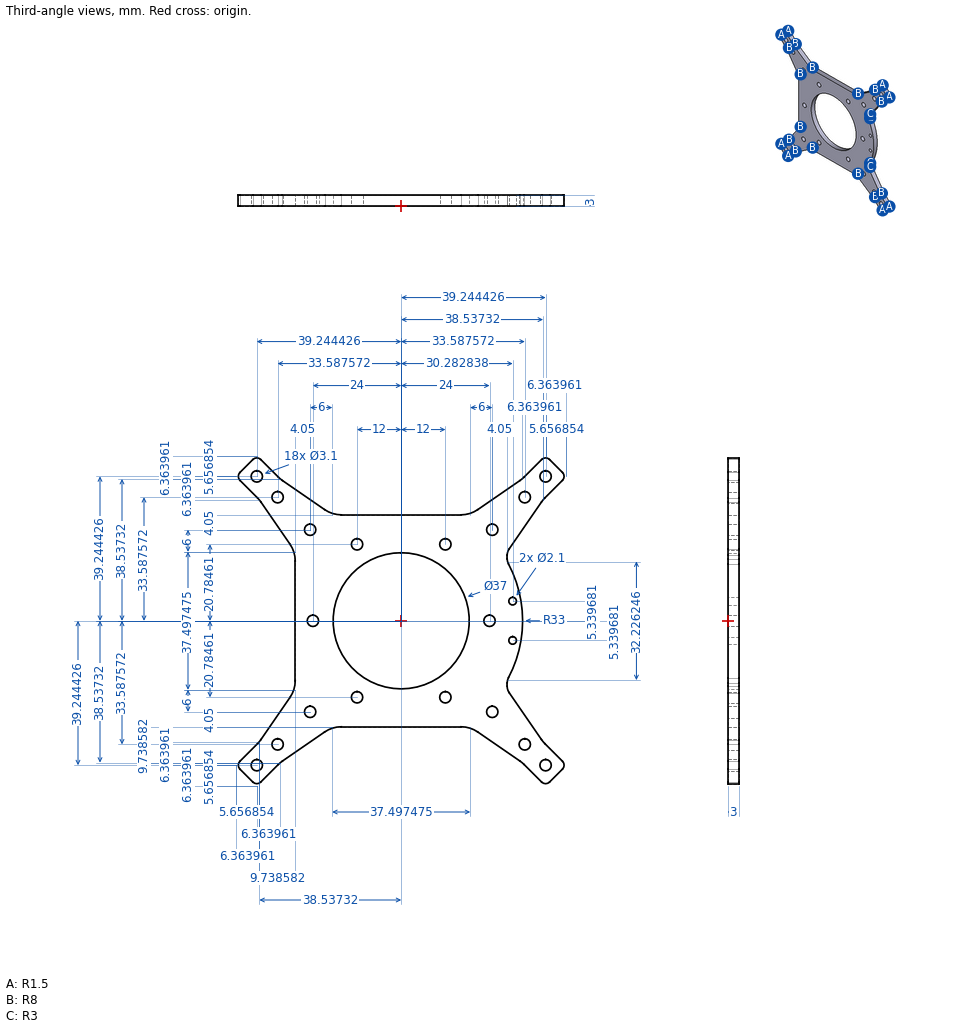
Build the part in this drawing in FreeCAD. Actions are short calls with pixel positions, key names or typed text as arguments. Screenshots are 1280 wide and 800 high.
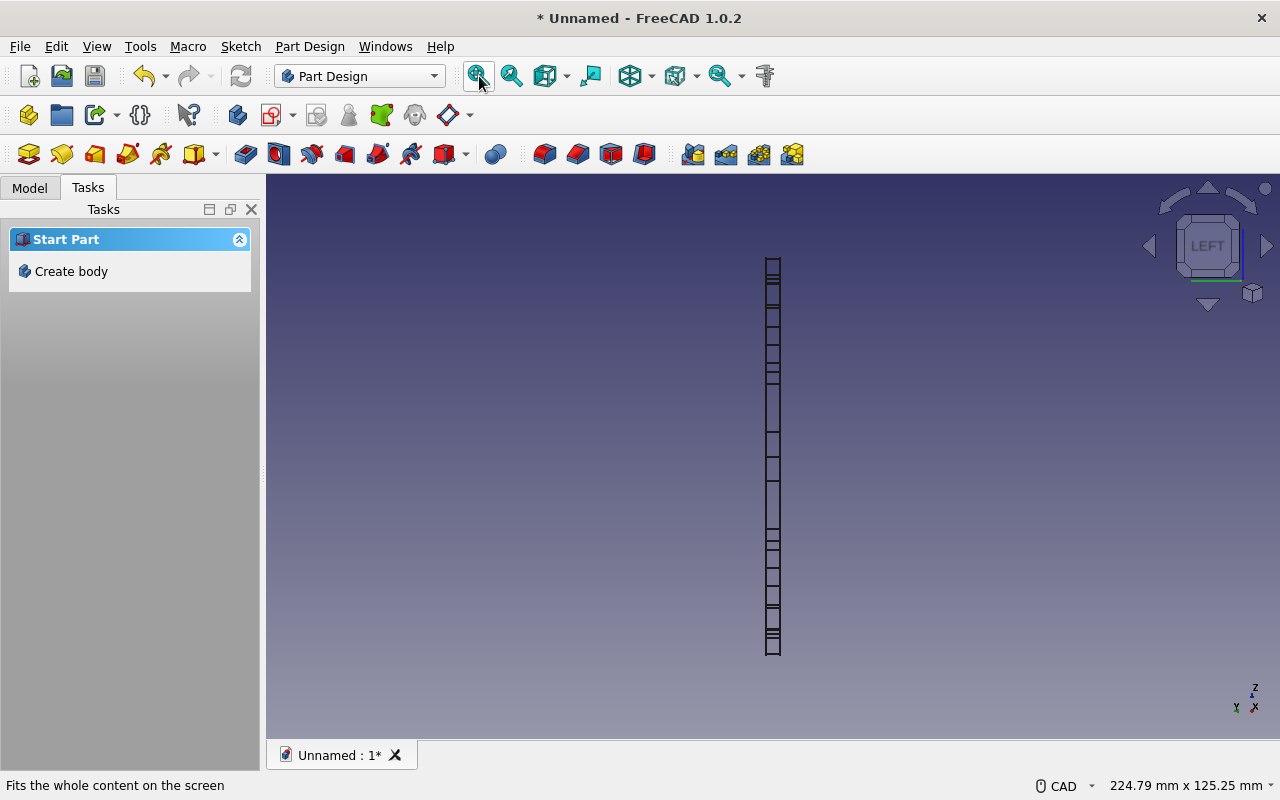
key(0)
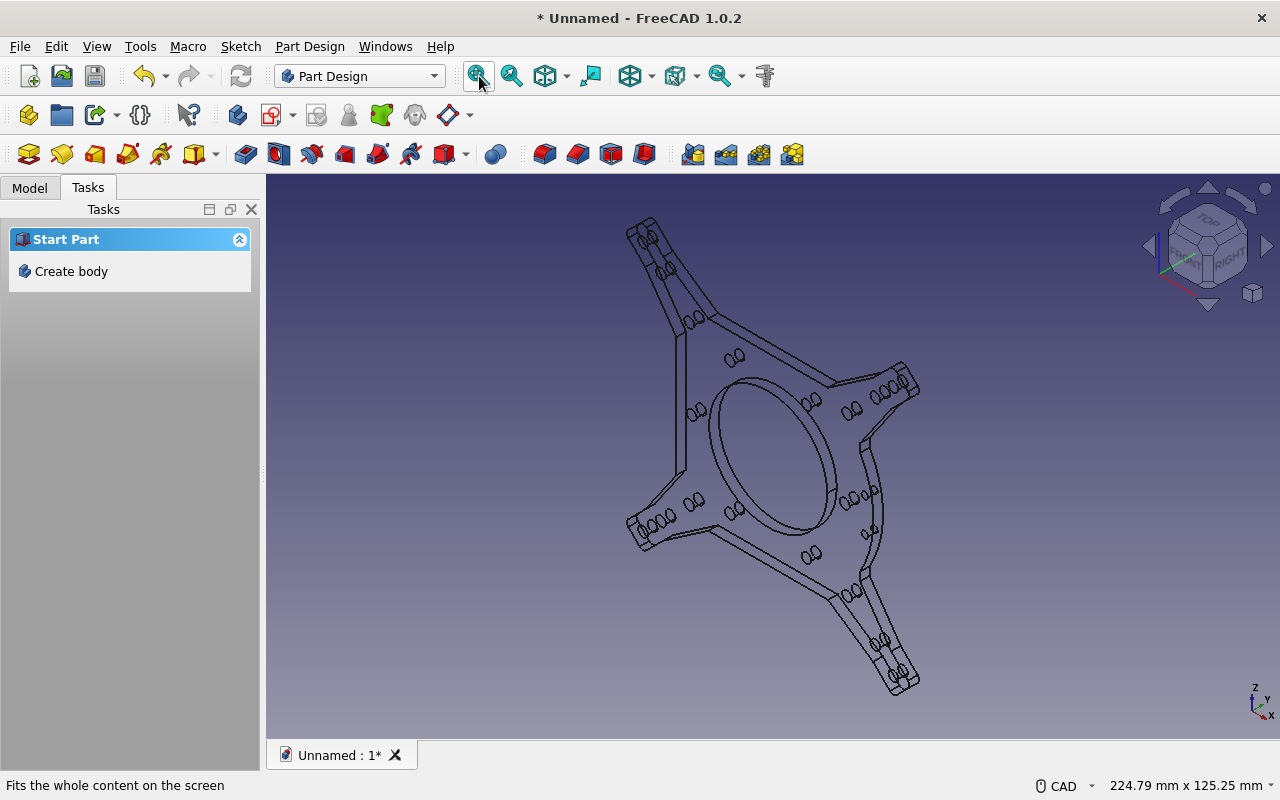
click(834, 596)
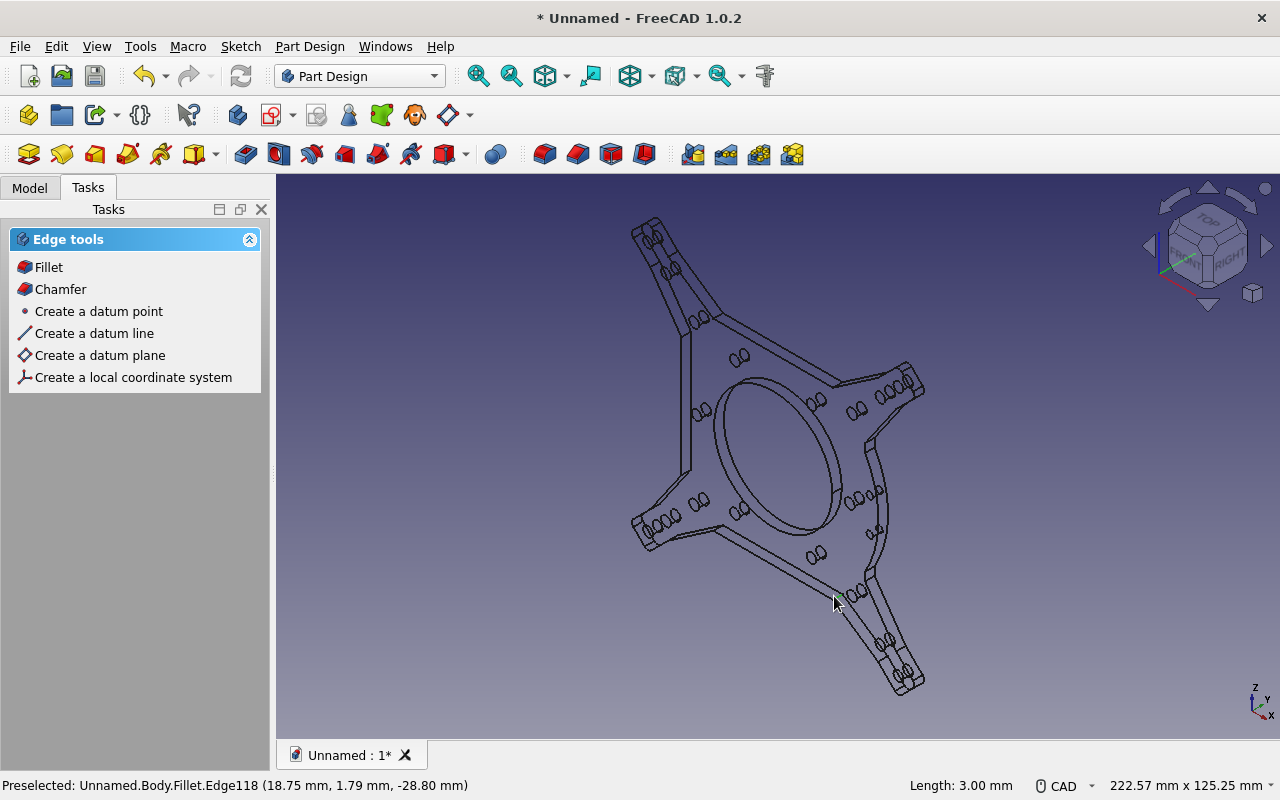
click(884, 657, ctrl)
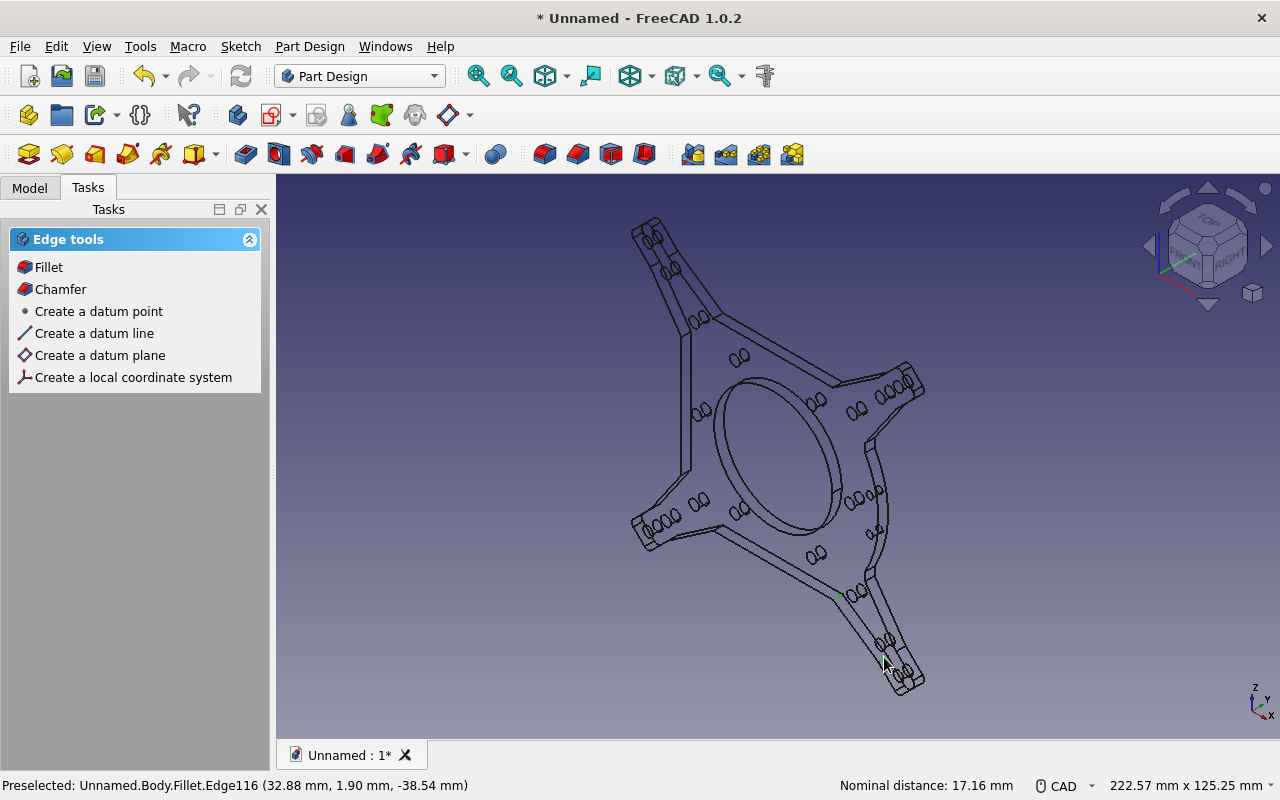
click(902, 647, ctrl)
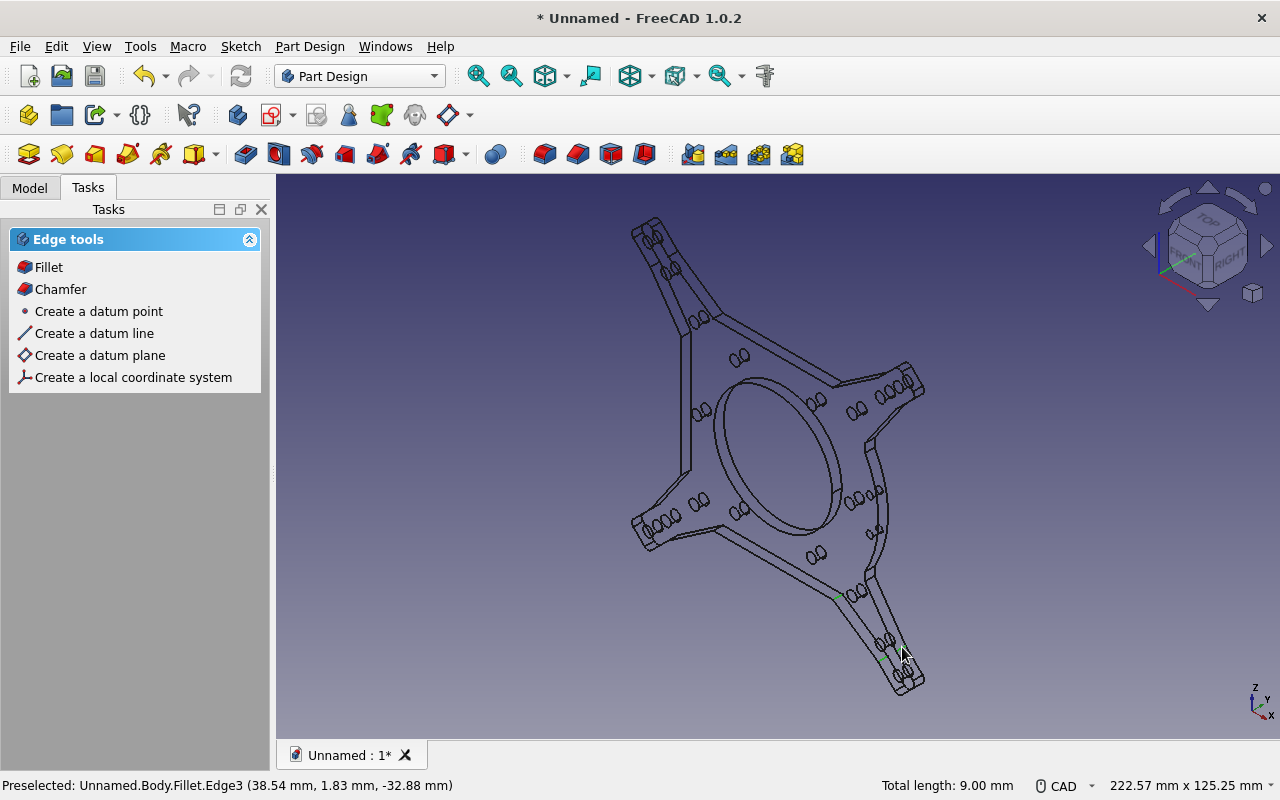
click(720, 314, ctrl)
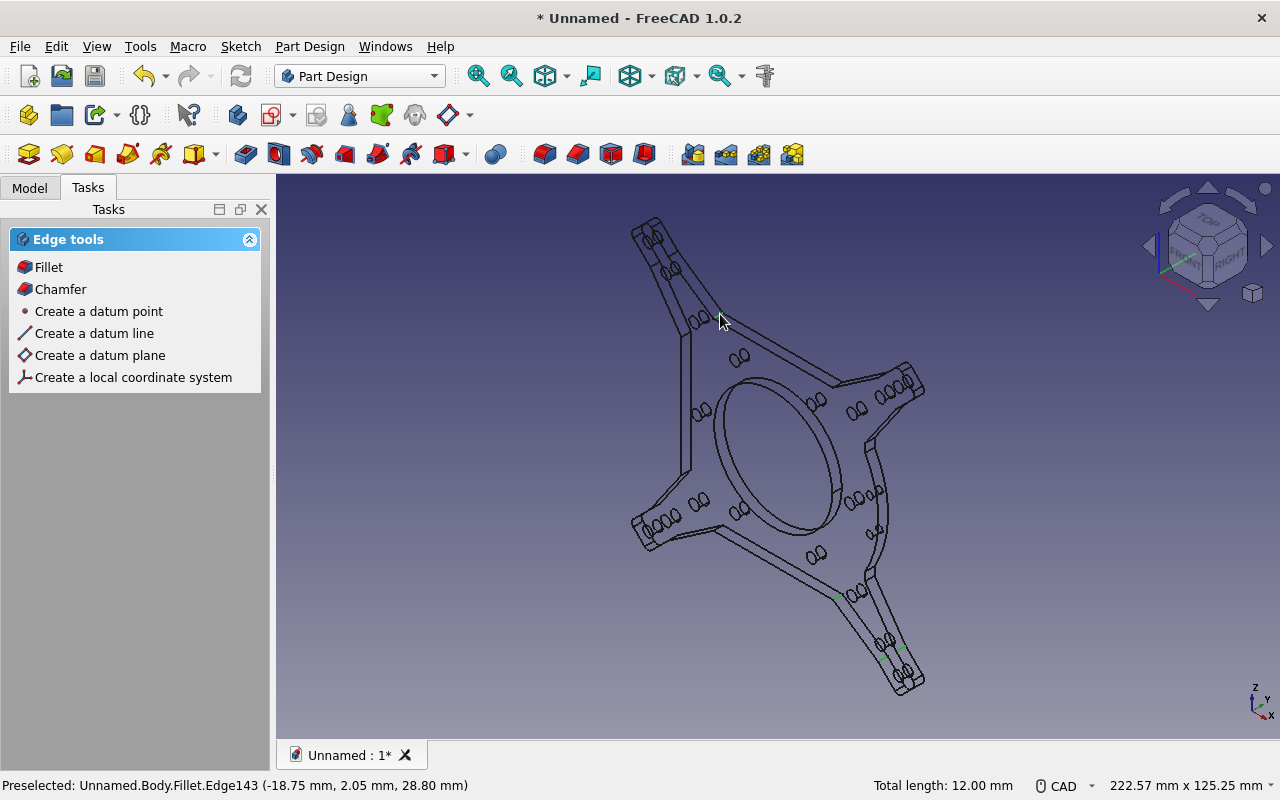
click(674, 252, ctrl)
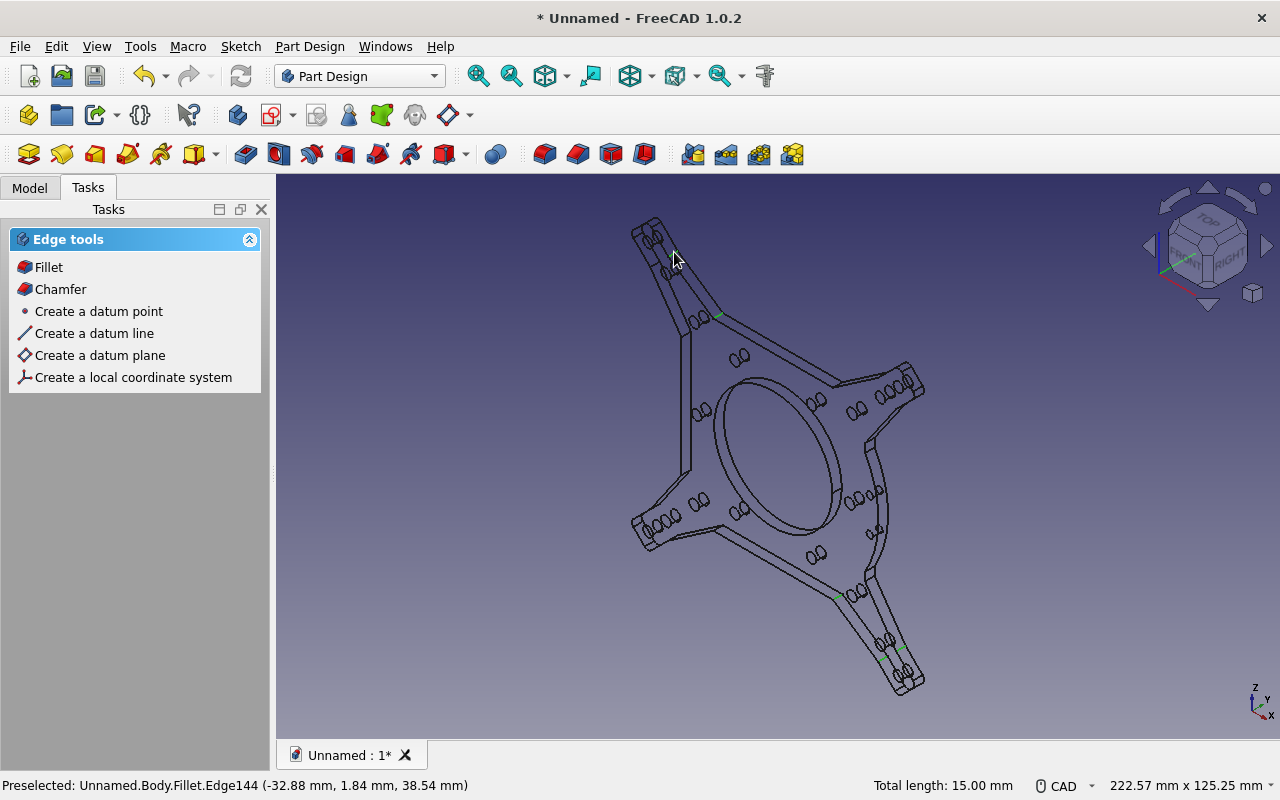
click(656, 263, ctrl)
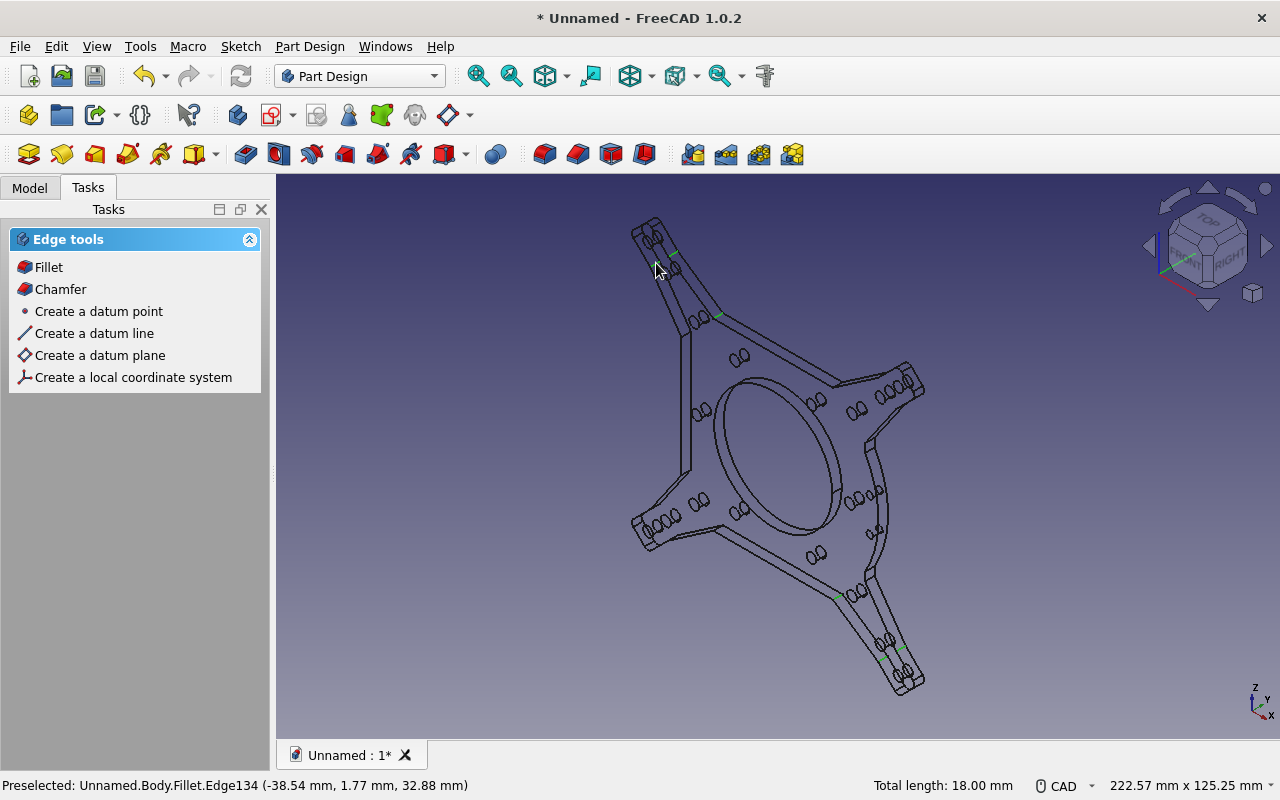
click(687, 333, ctrl)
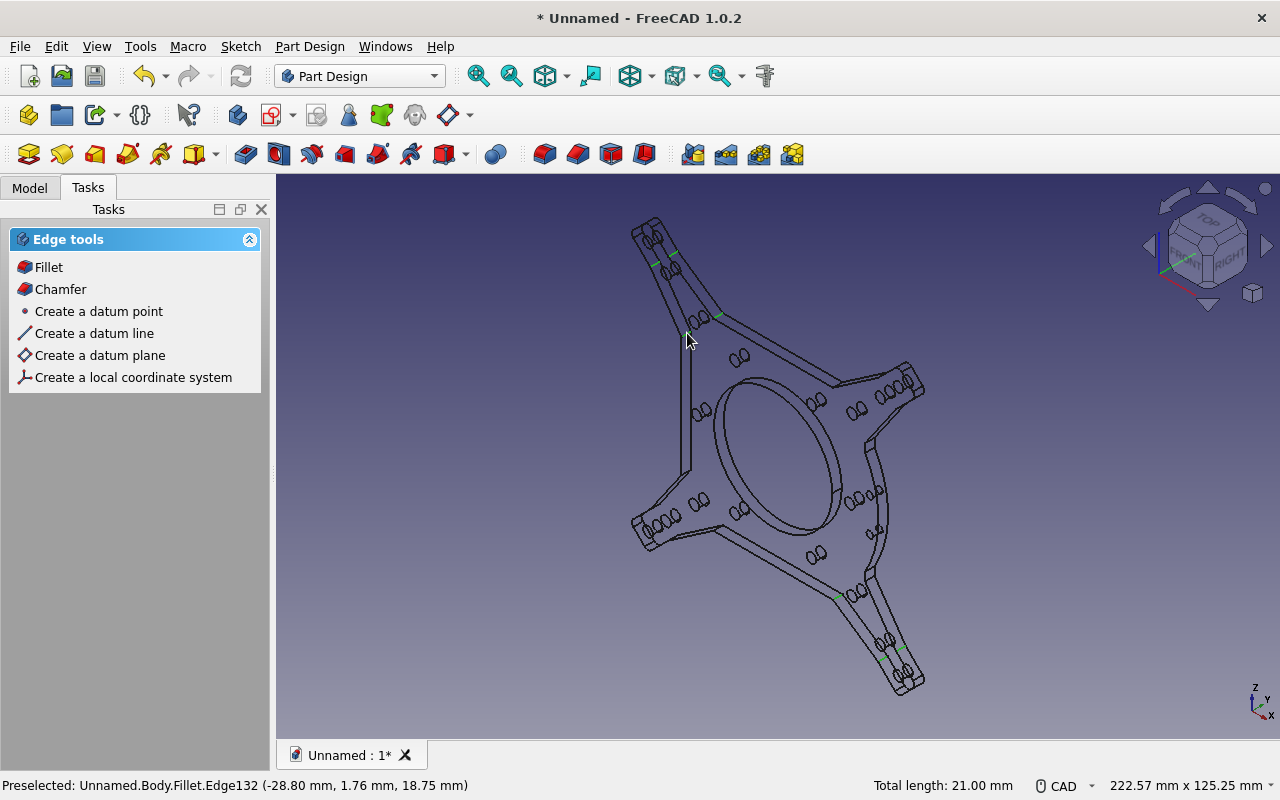
click(688, 470, ctrl)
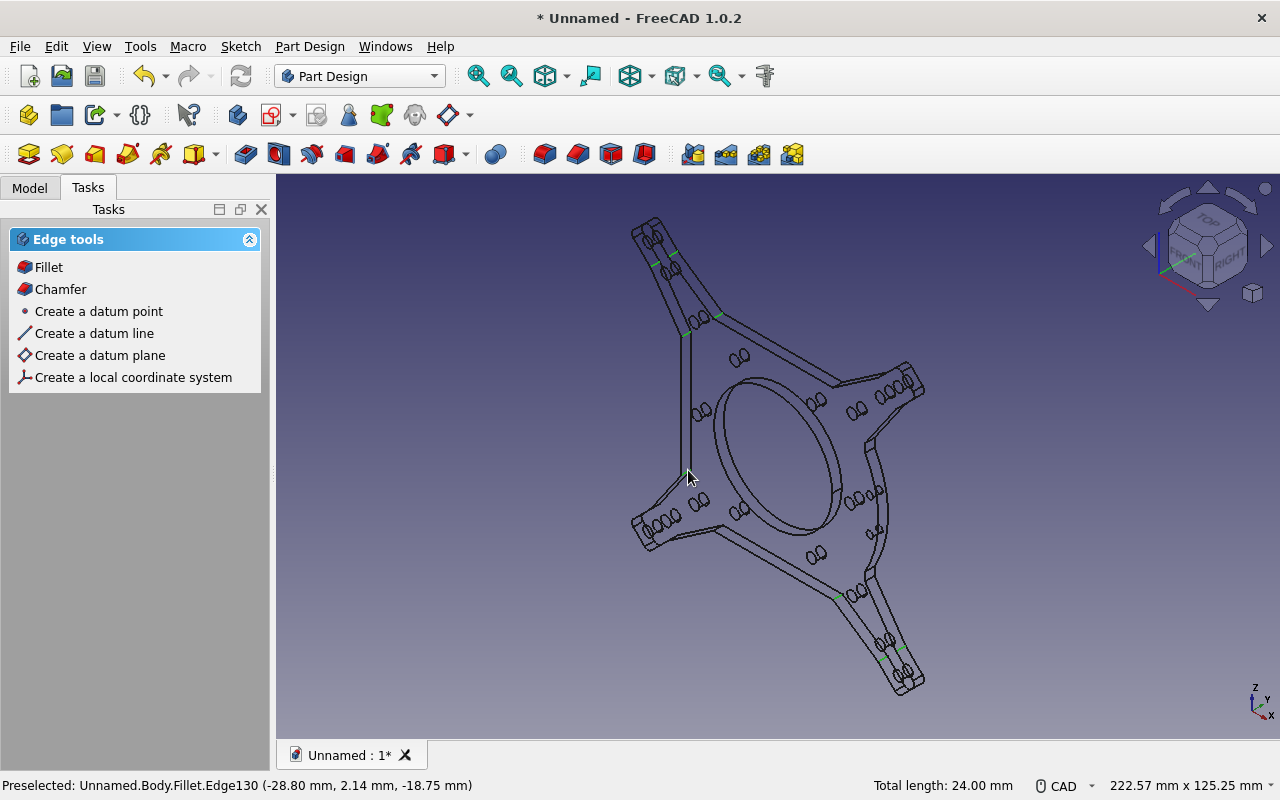
click(720, 526, ctrl)